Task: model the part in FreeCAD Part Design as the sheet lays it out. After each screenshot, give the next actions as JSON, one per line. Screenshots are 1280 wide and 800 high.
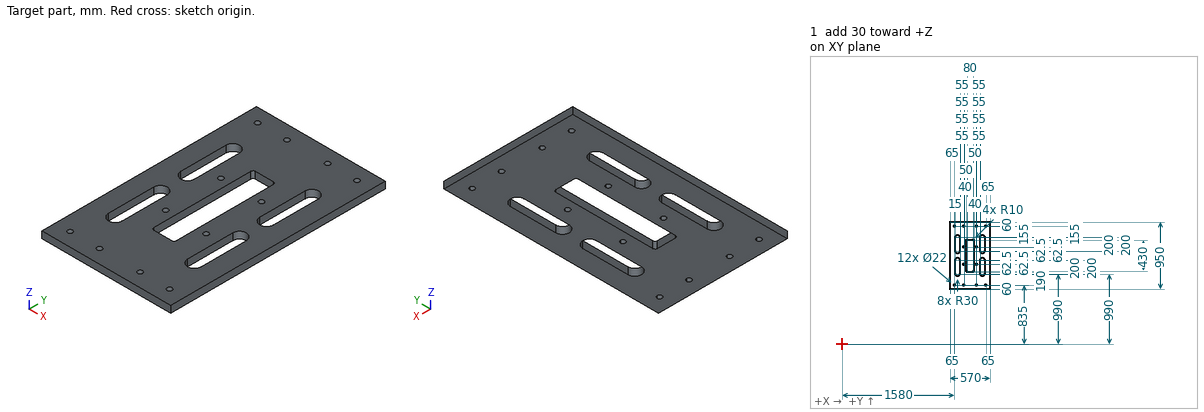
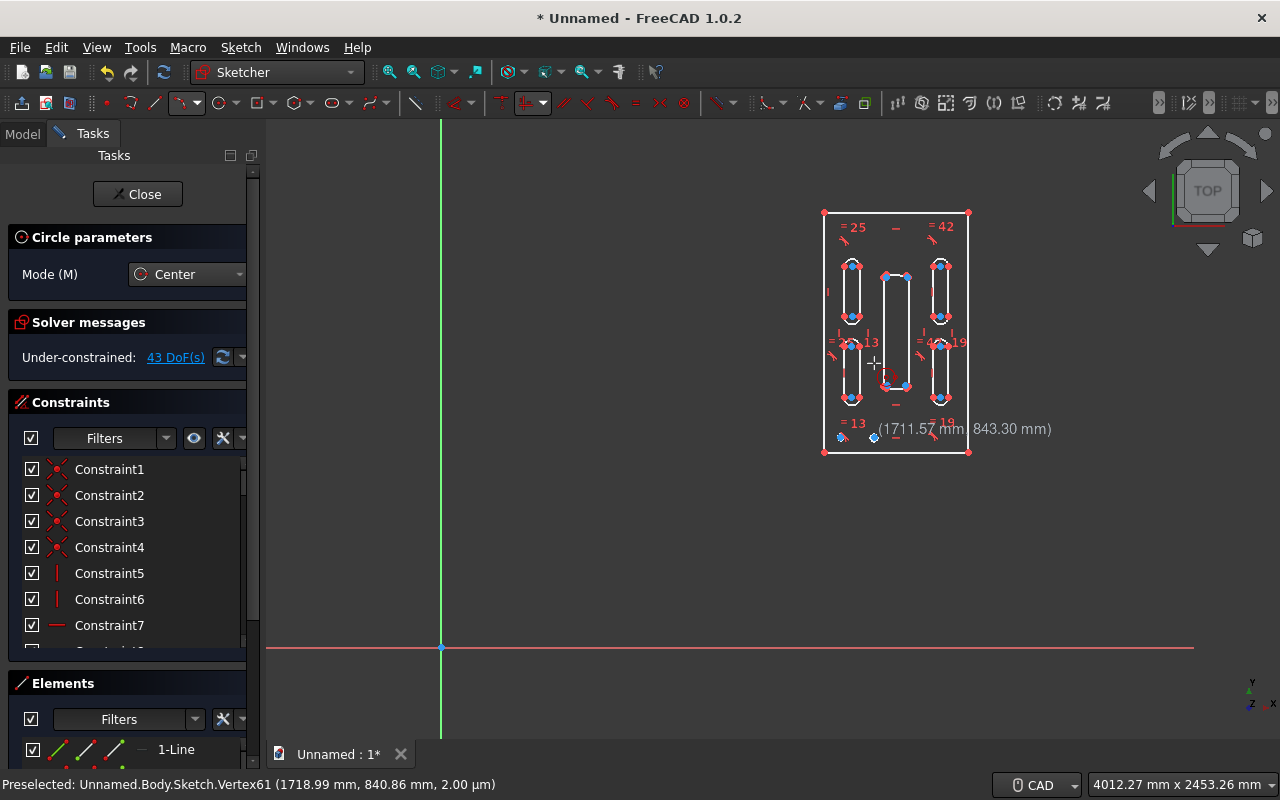
{"action": "scroll", "coordinate": [874, 363], "scroll_direction": "up", "scroll_amount": 3}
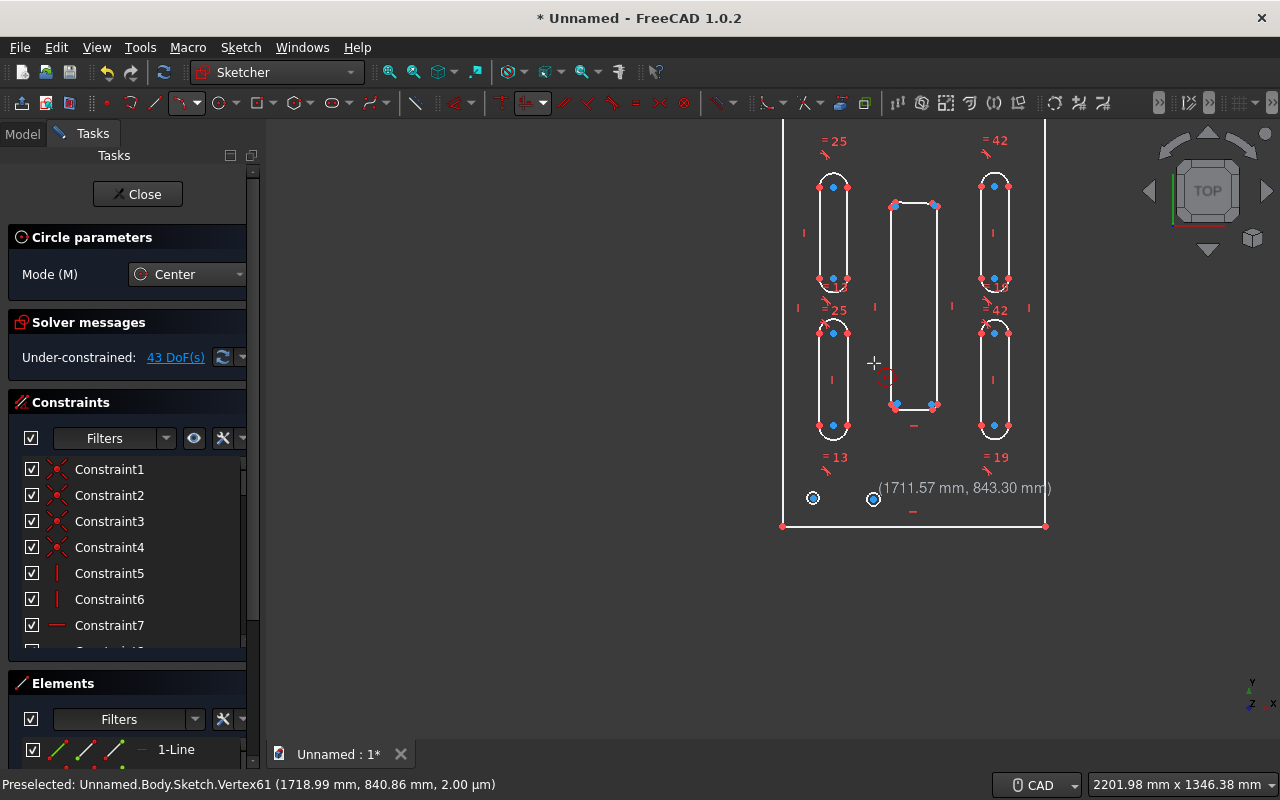
{"action": "left_click", "coordinate": [873, 362]}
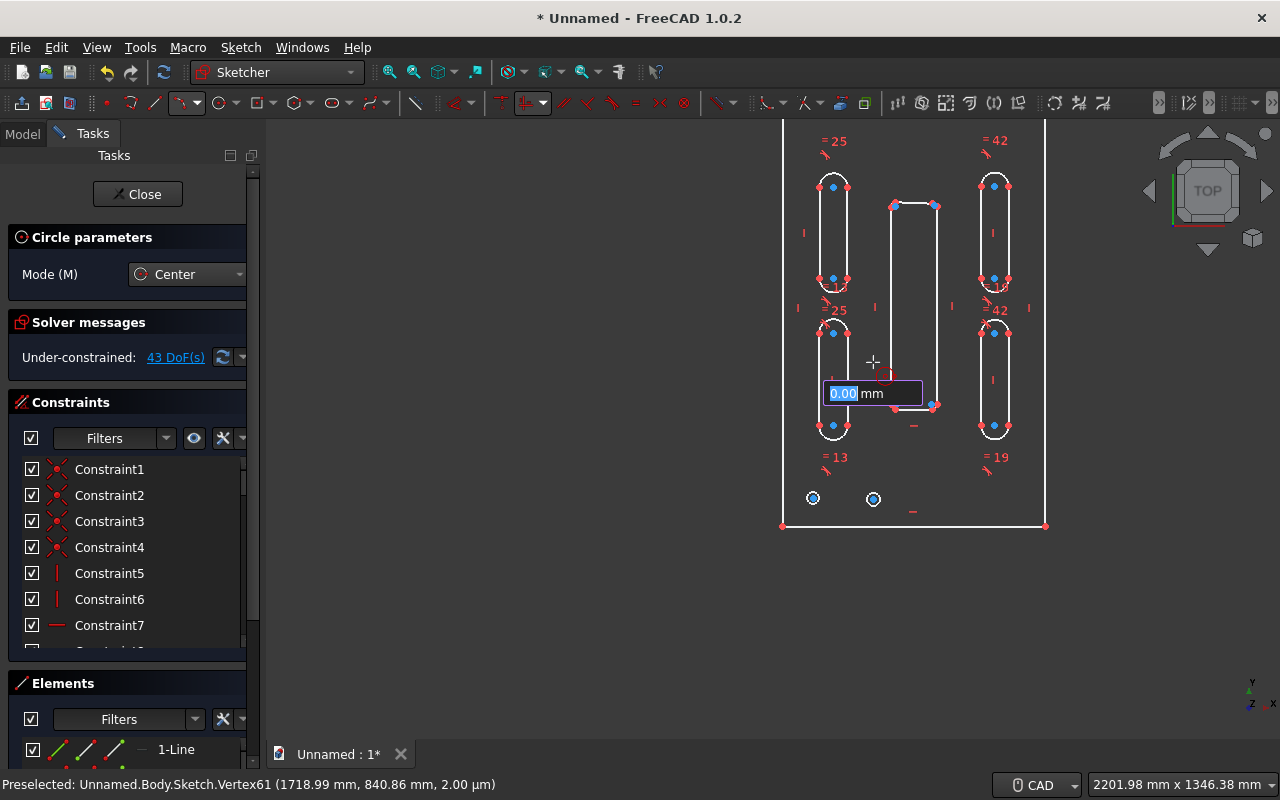
{"action": "scroll", "coordinate": [876, 358], "scroll_direction": "up", "scroll_amount": 6}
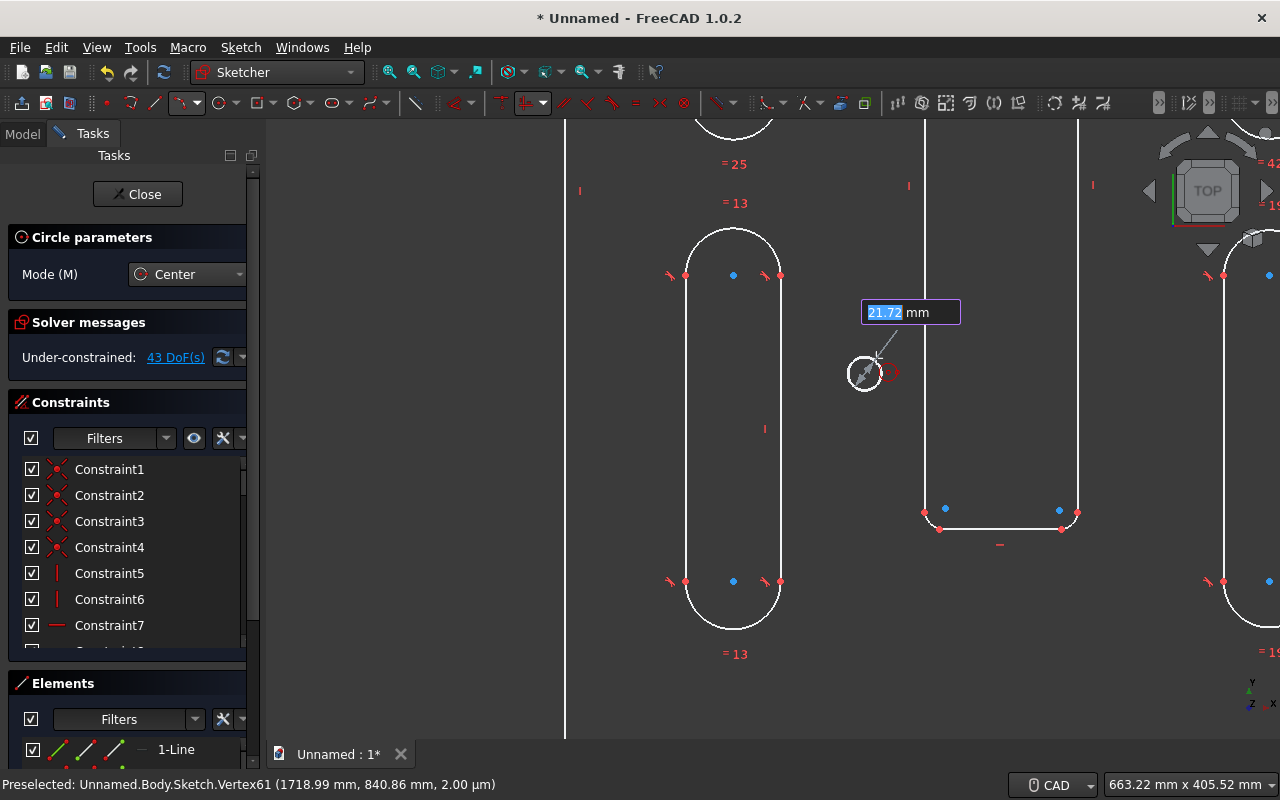
{"action": "left_click", "coordinate": [876, 358]}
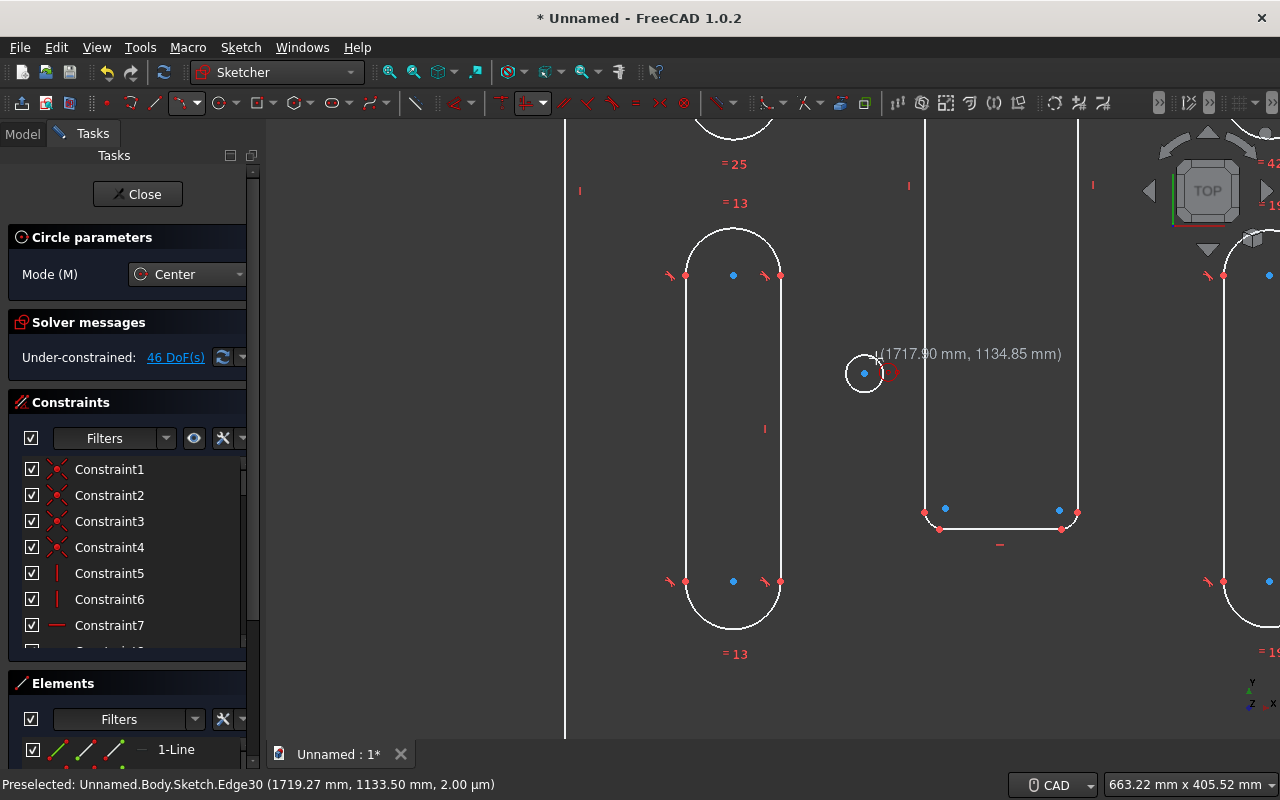
{"action": "scroll", "coordinate": [875, 360], "scroll_direction": "down", "scroll_amount": 9}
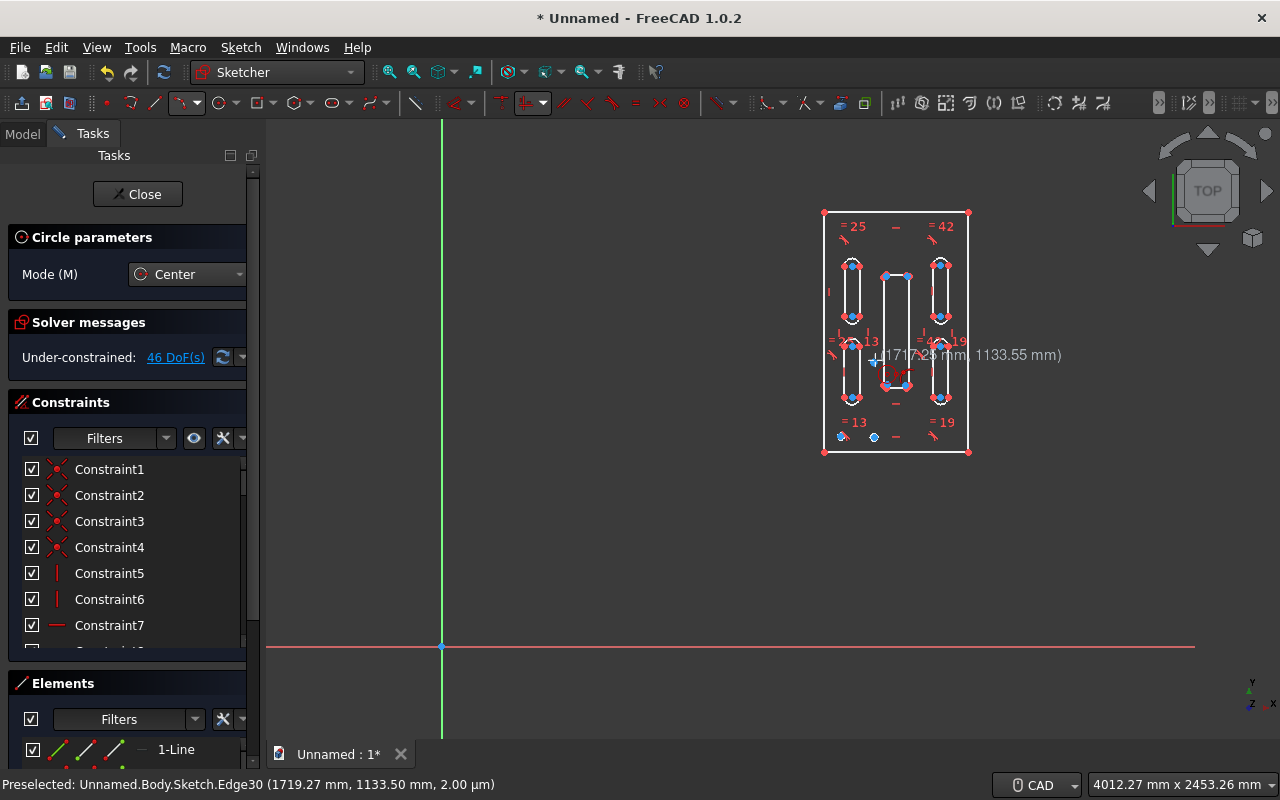
{"action": "scroll", "coordinate": [919, 436], "scroll_direction": "up", "scroll_amount": 11}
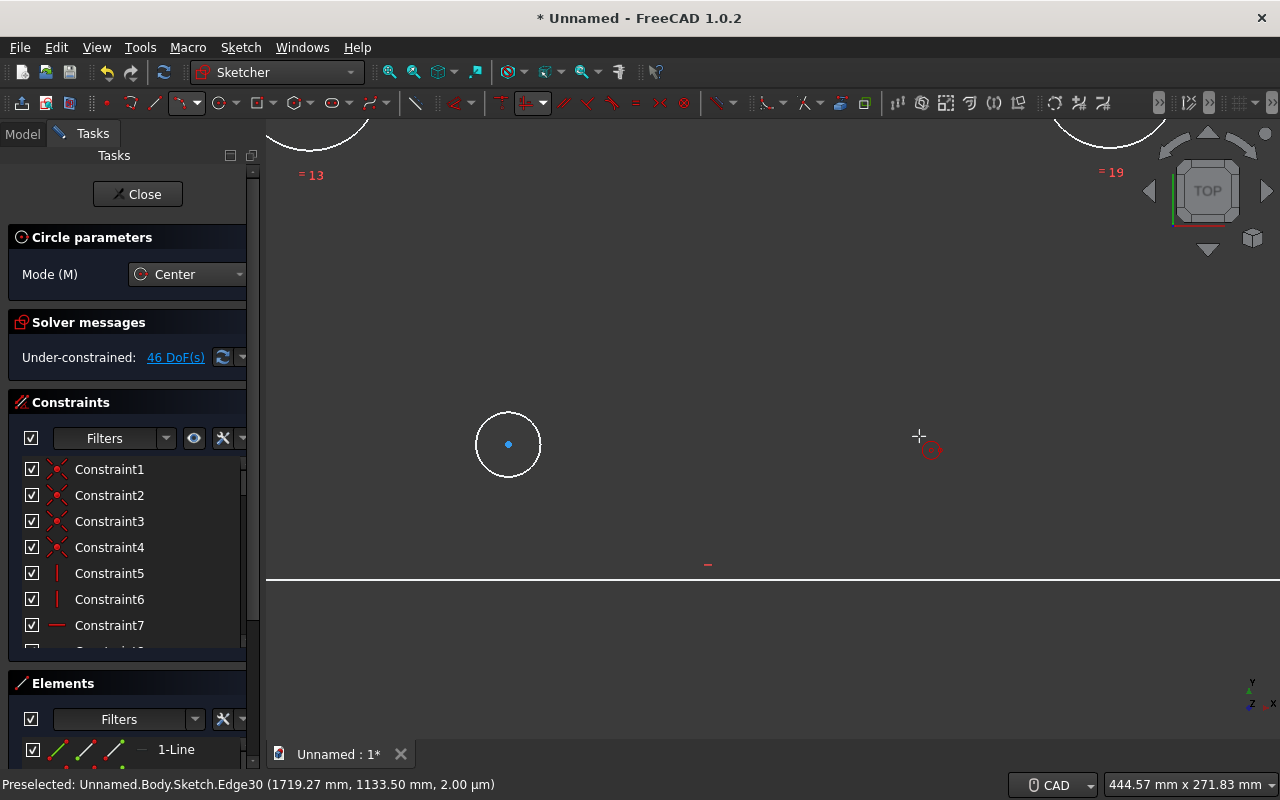
{"action": "scroll", "coordinate": [919, 437], "scroll_direction": "down", "scroll_amount": 11}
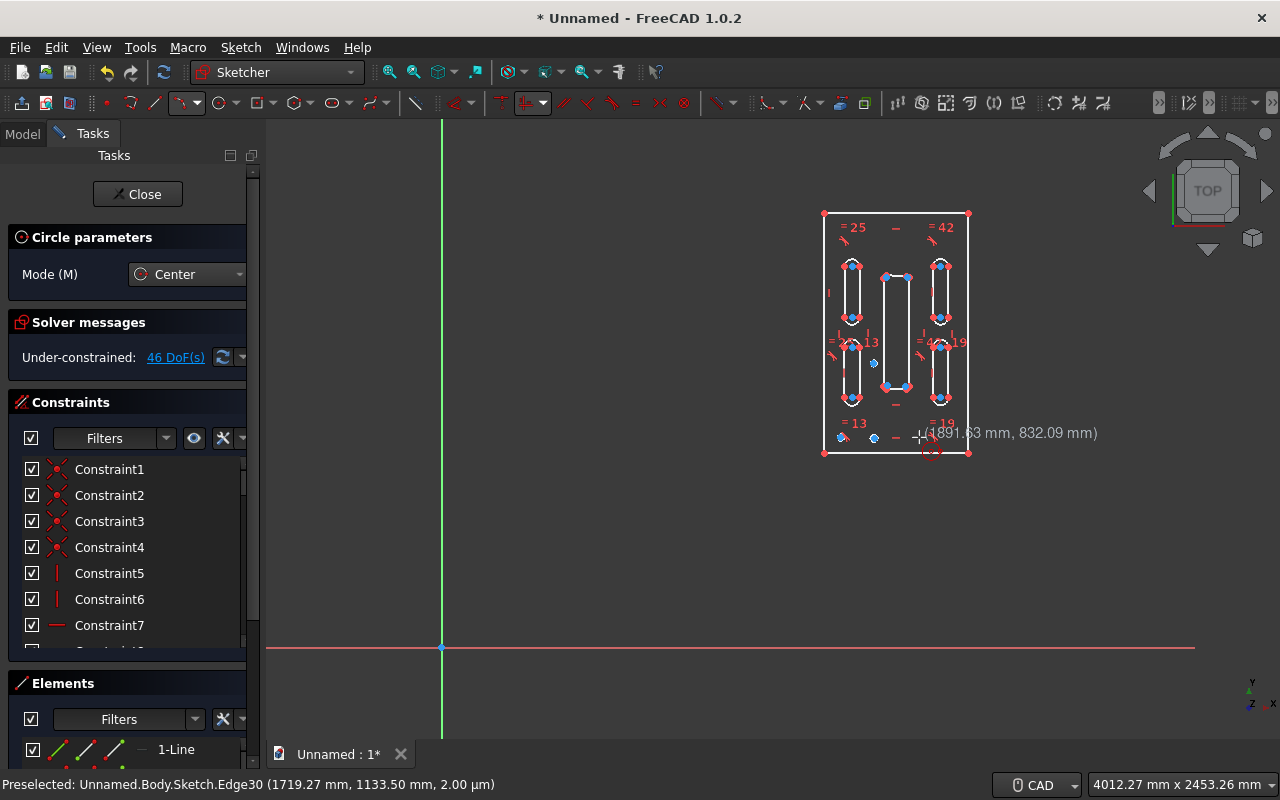
{"action": "left_click", "coordinate": [919, 437]}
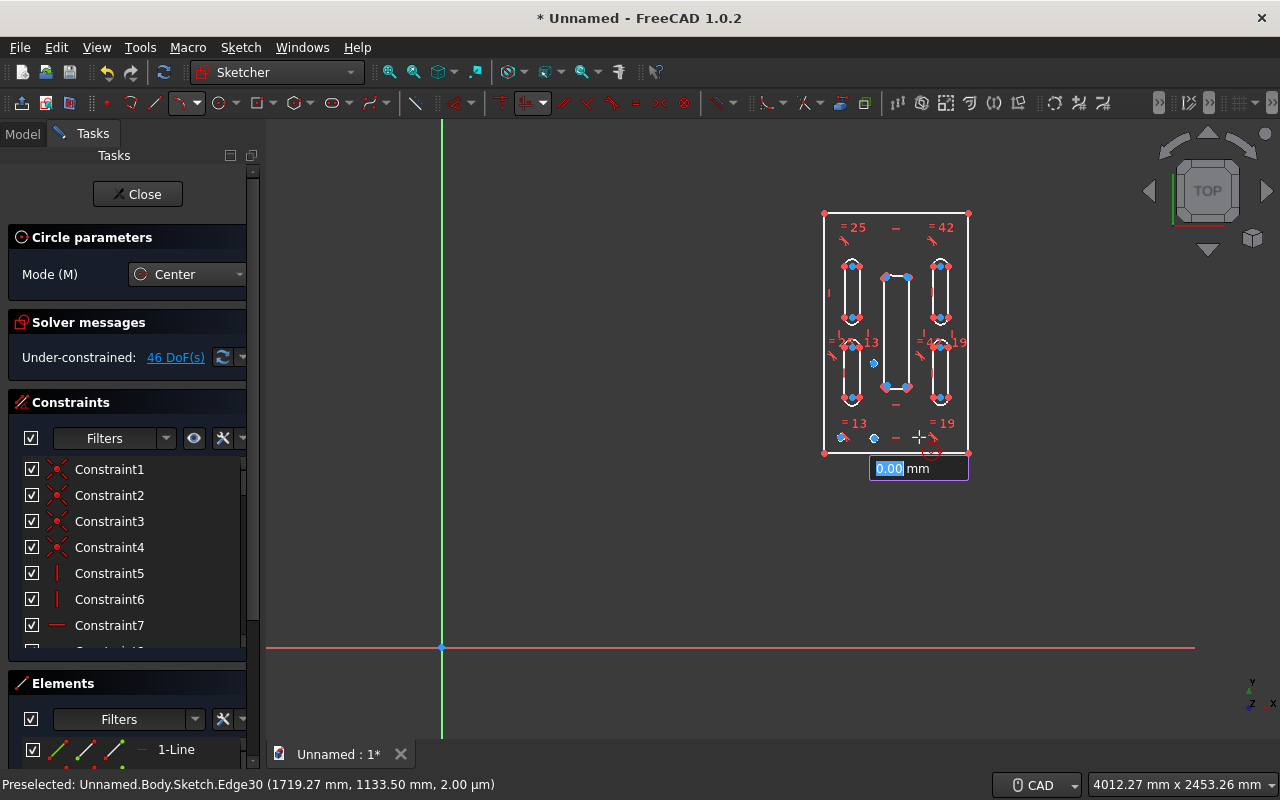
{"action": "scroll", "coordinate": [921, 435], "scroll_direction": "up", "scroll_amount": 9}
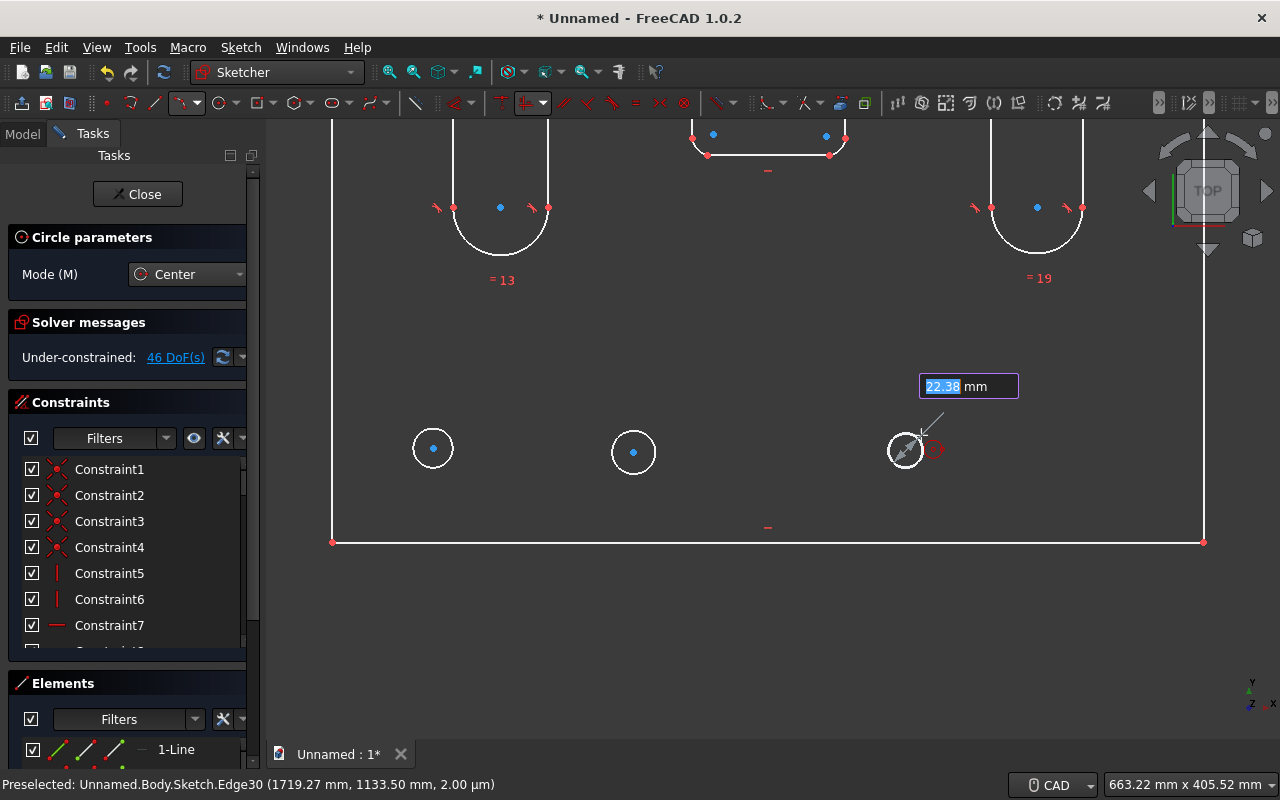
{"action": "left_click", "coordinate": [919, 432]}